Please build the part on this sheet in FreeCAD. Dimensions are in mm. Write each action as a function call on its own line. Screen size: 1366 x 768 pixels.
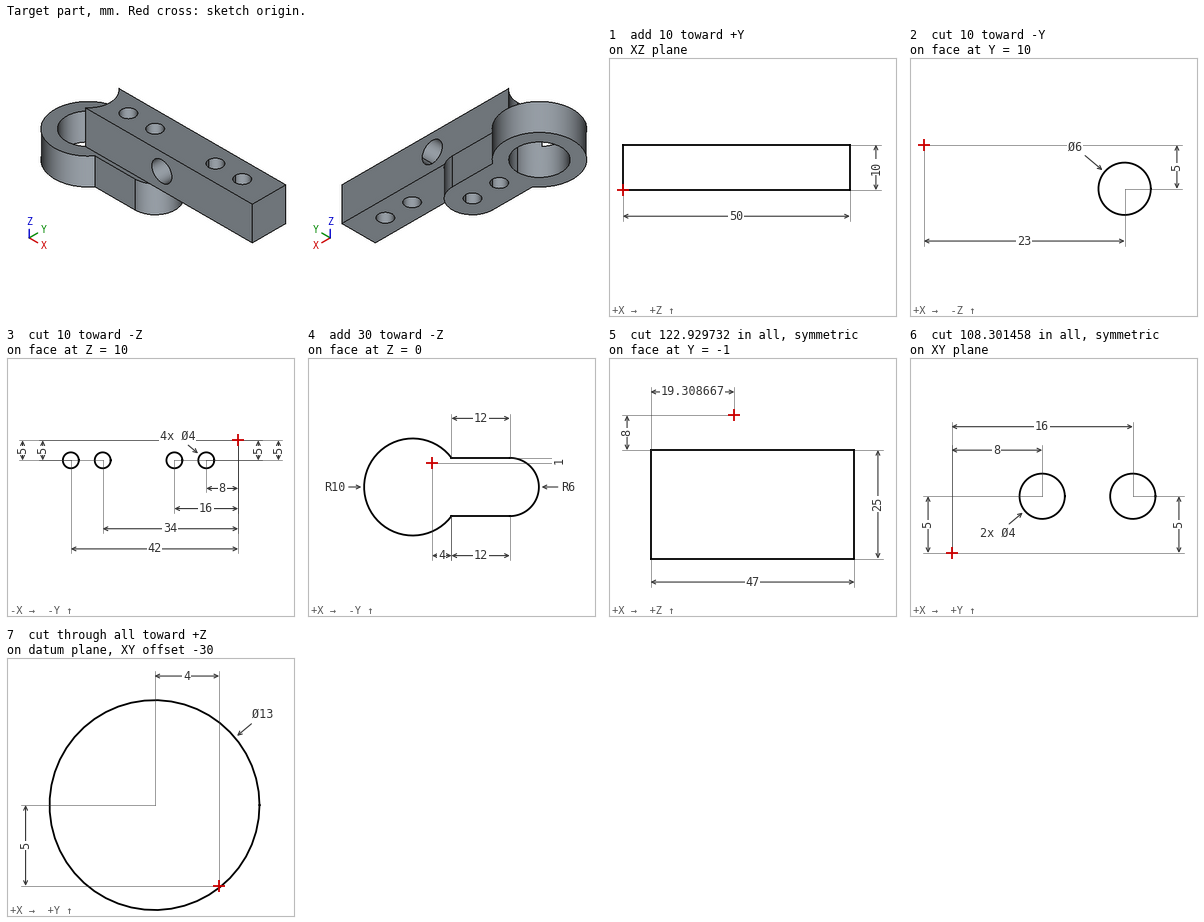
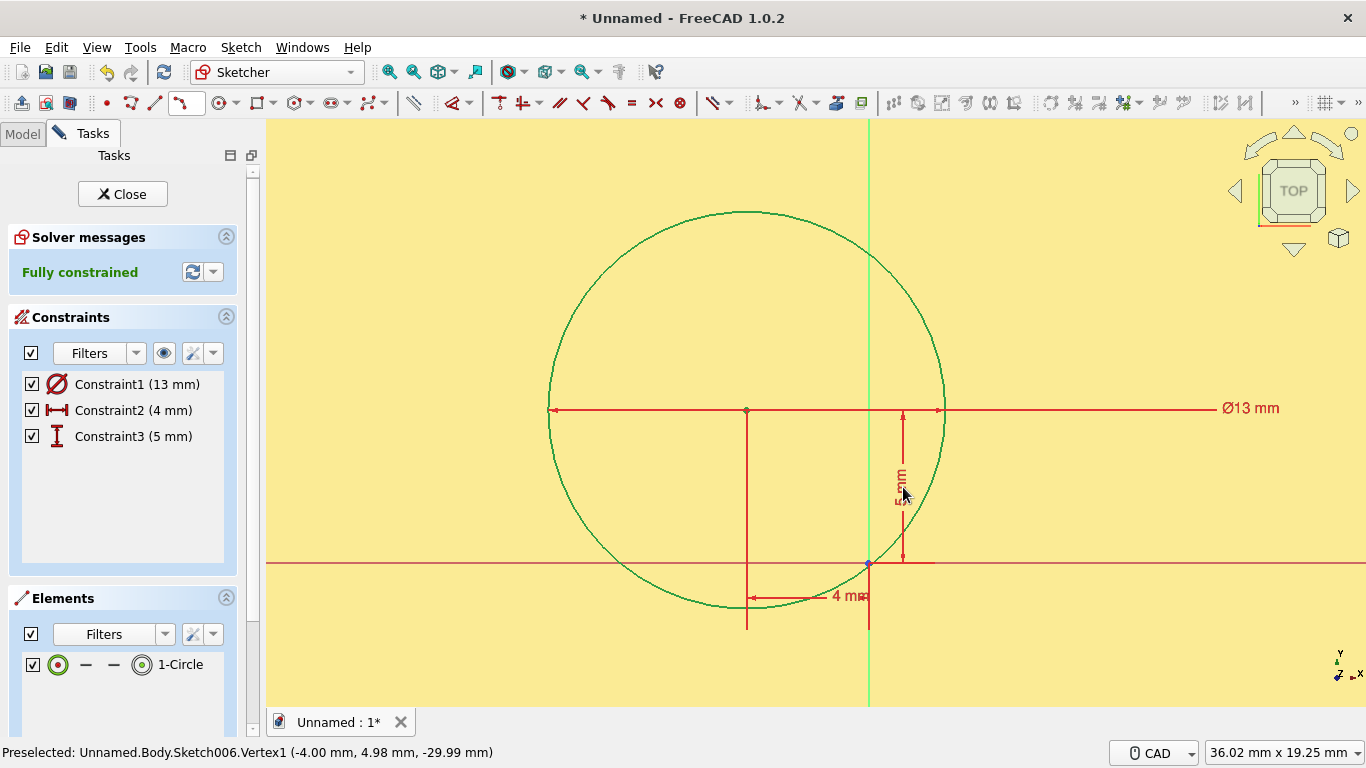
click(123, 194)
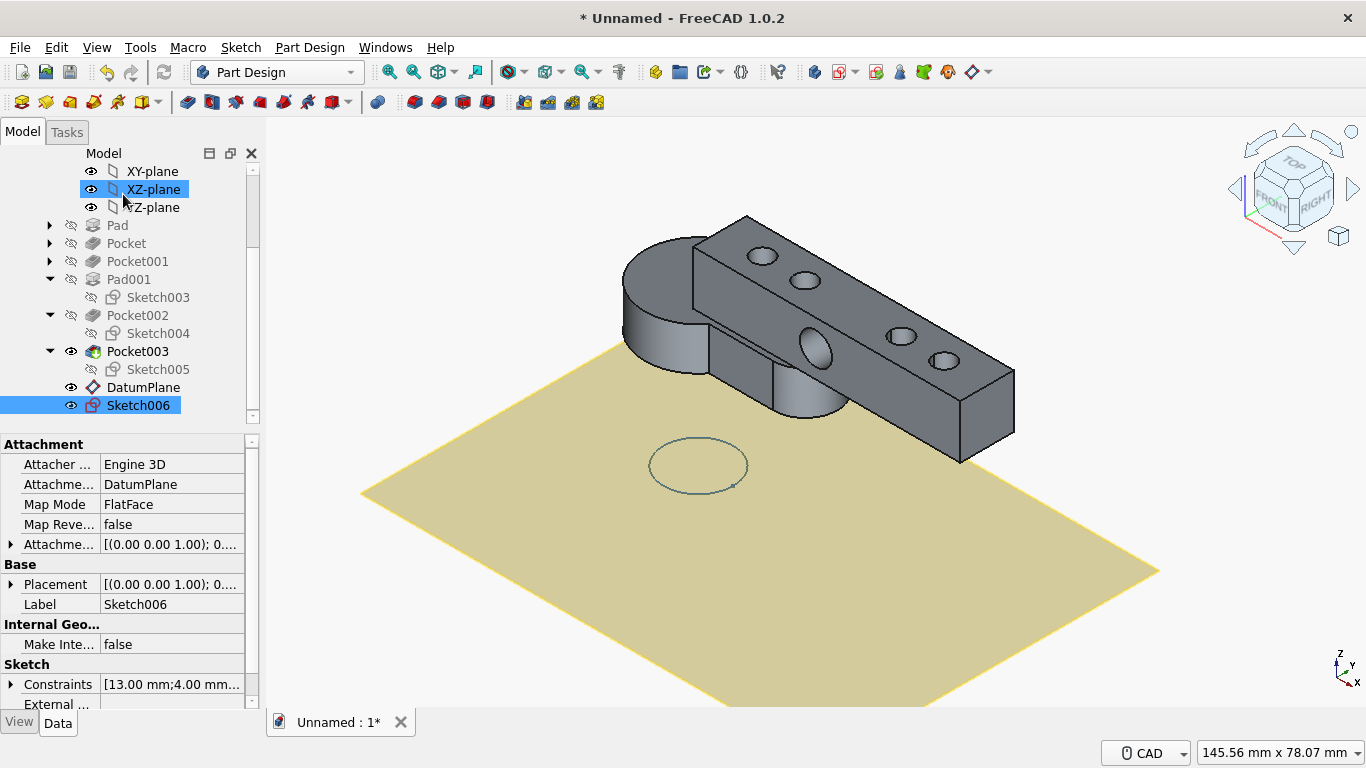
click(188, 102)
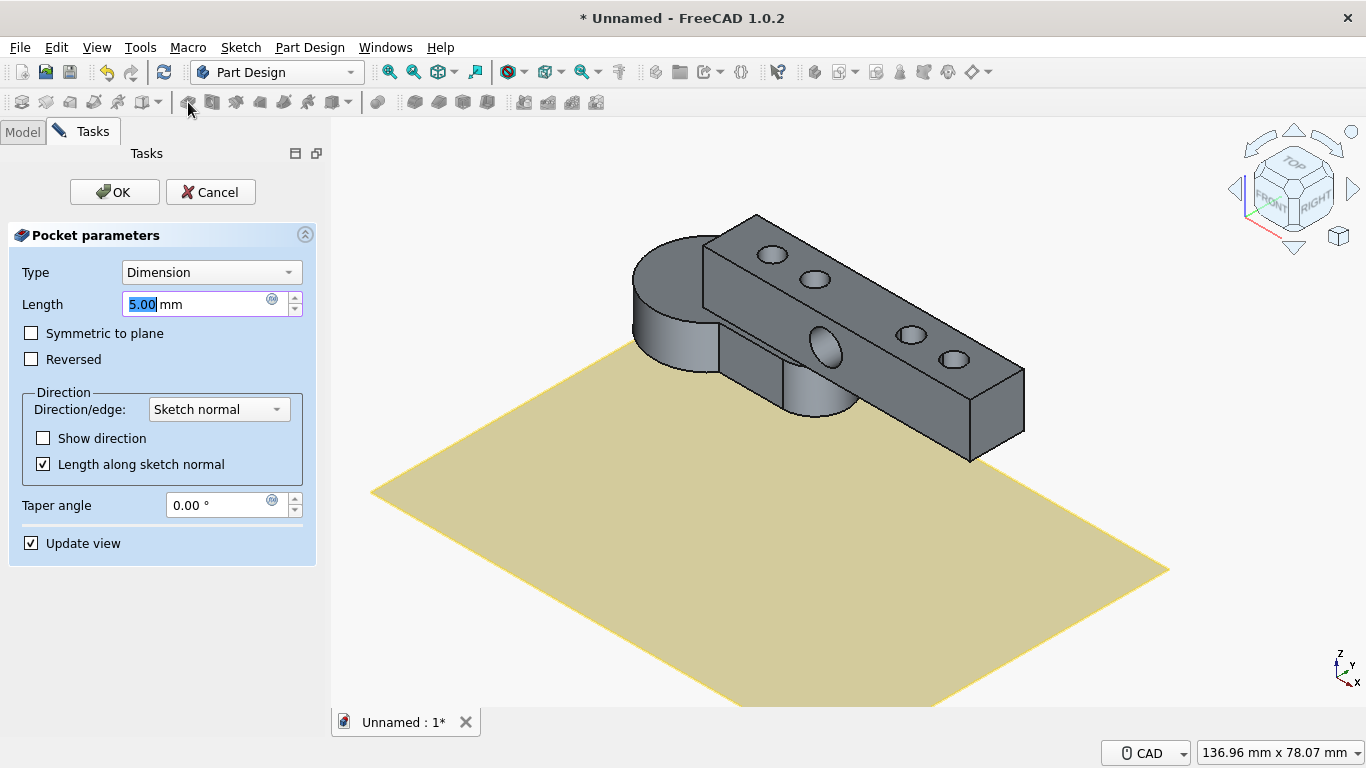
click(212, 272)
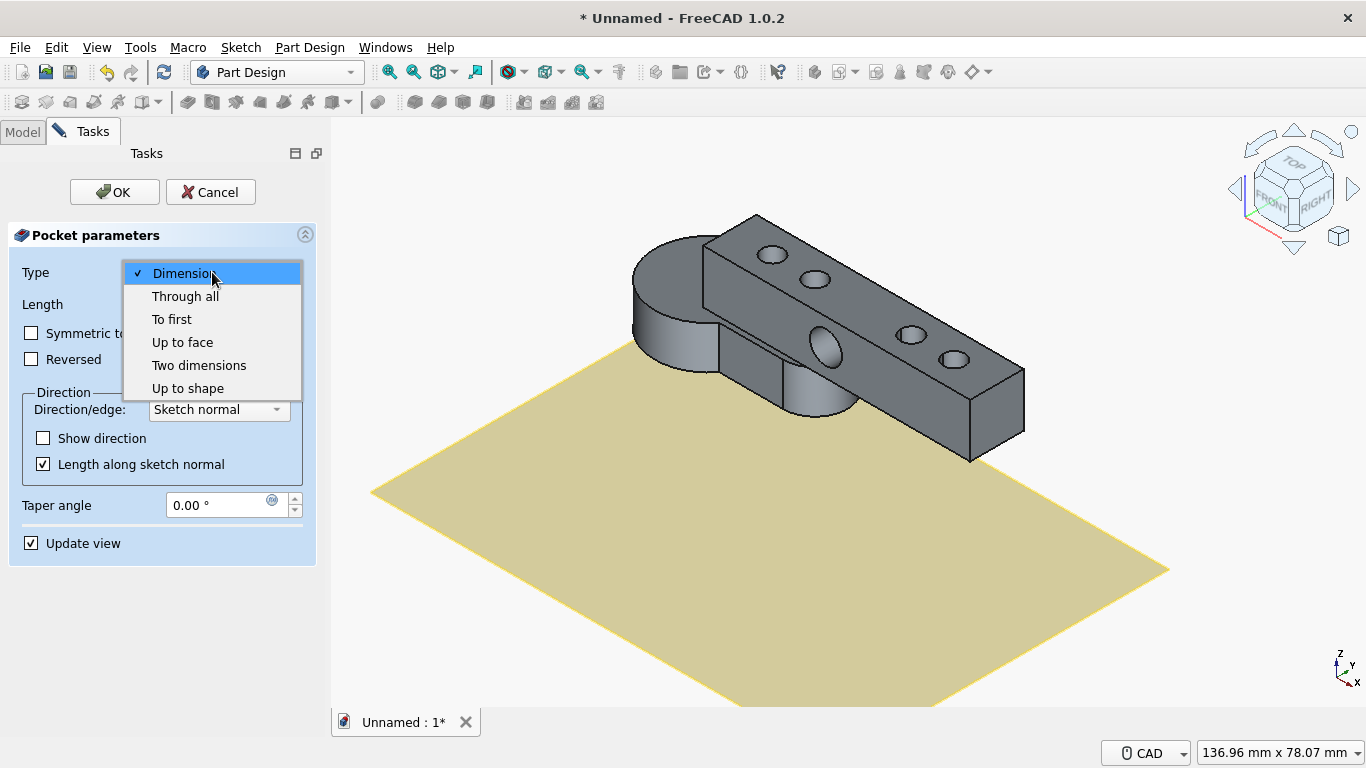
click(212, 296)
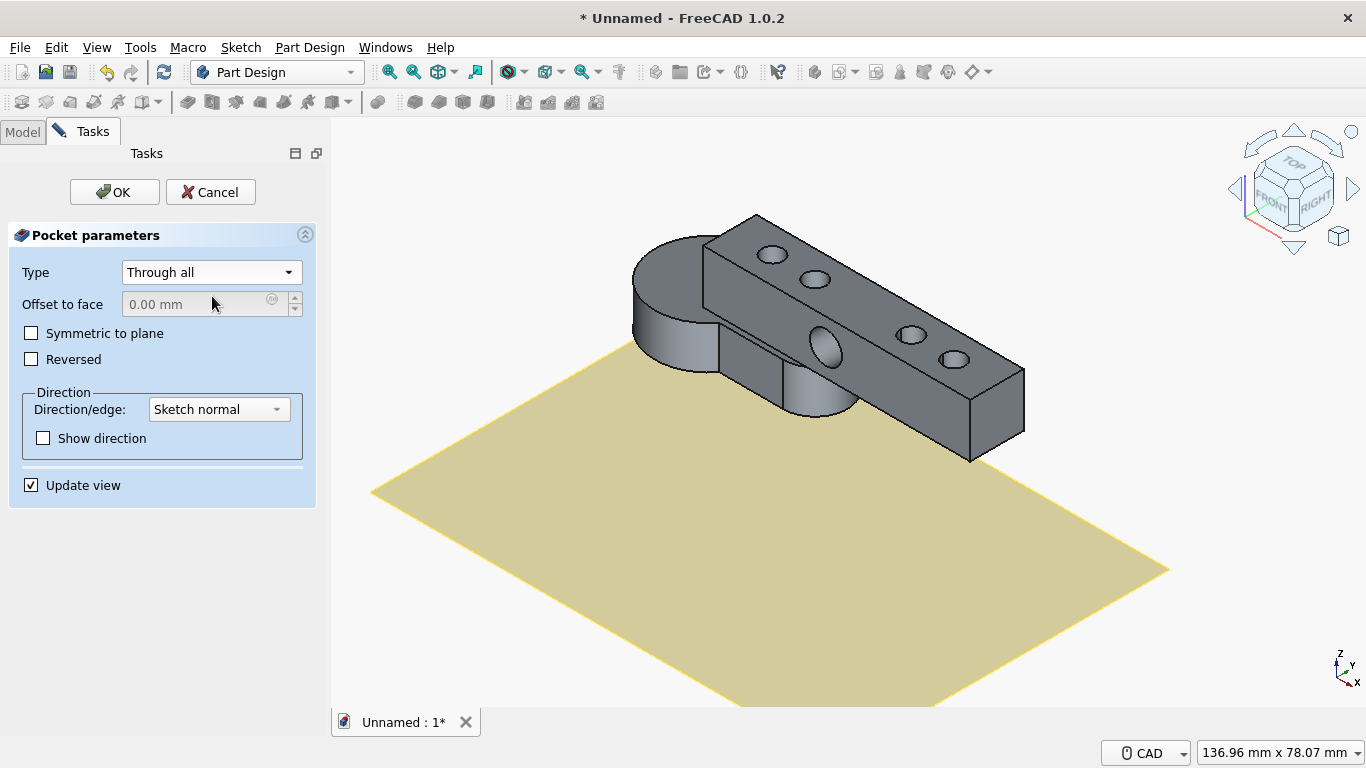
click(30, 359)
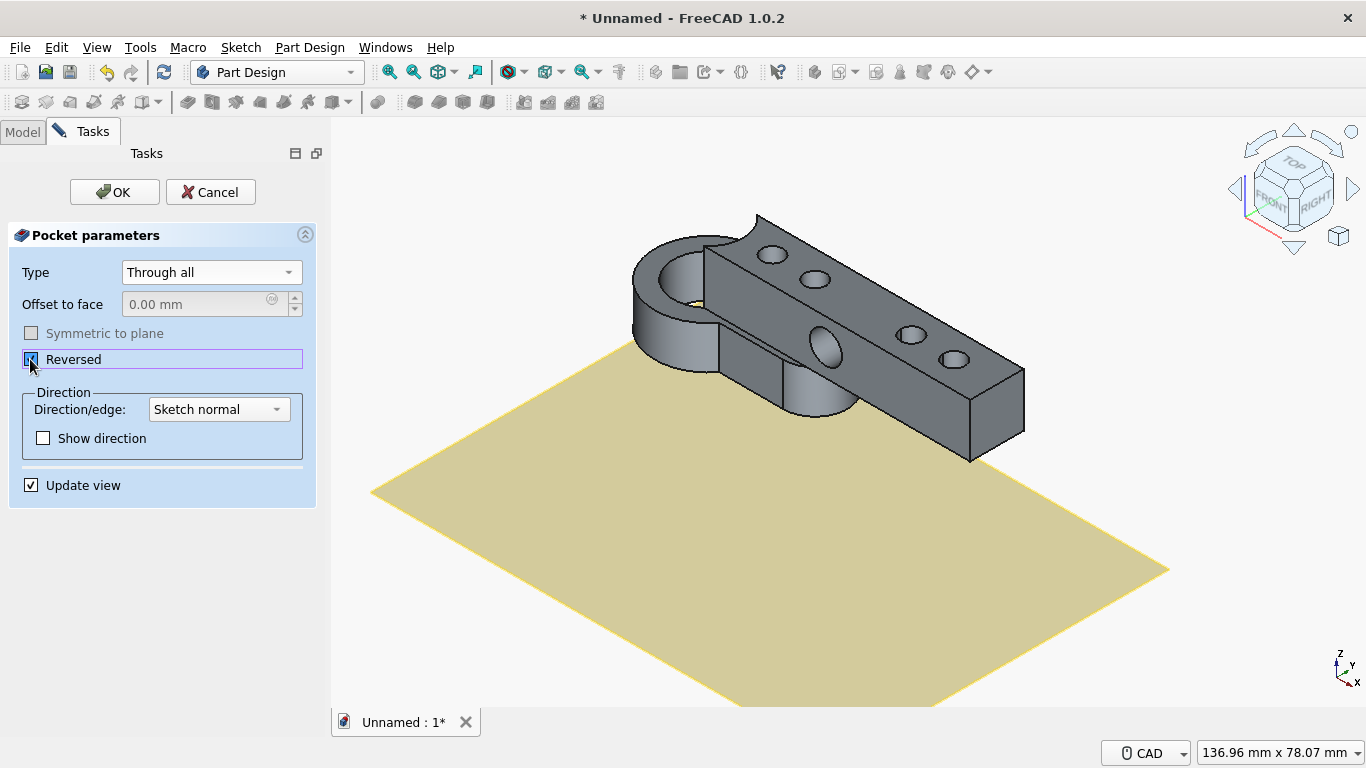
click(115, 192)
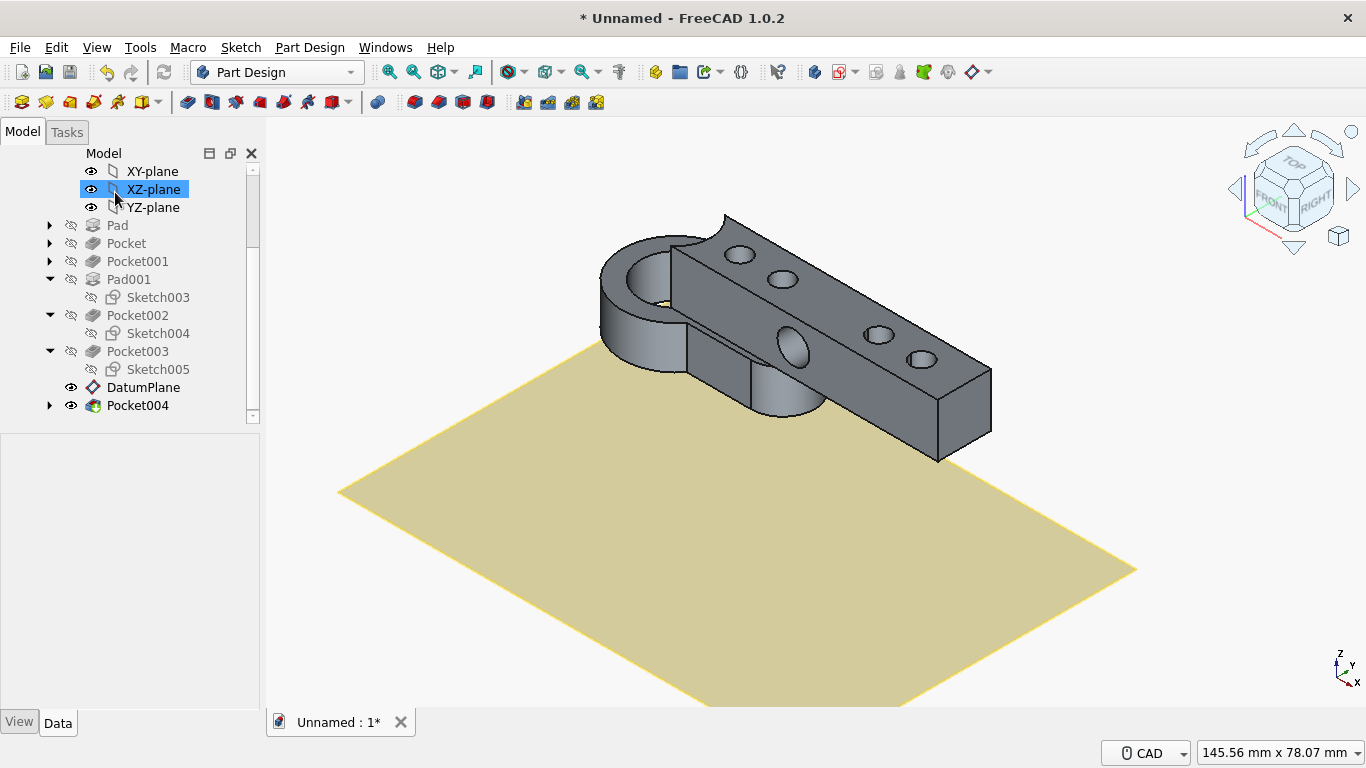
click(116, 387)
key(space)